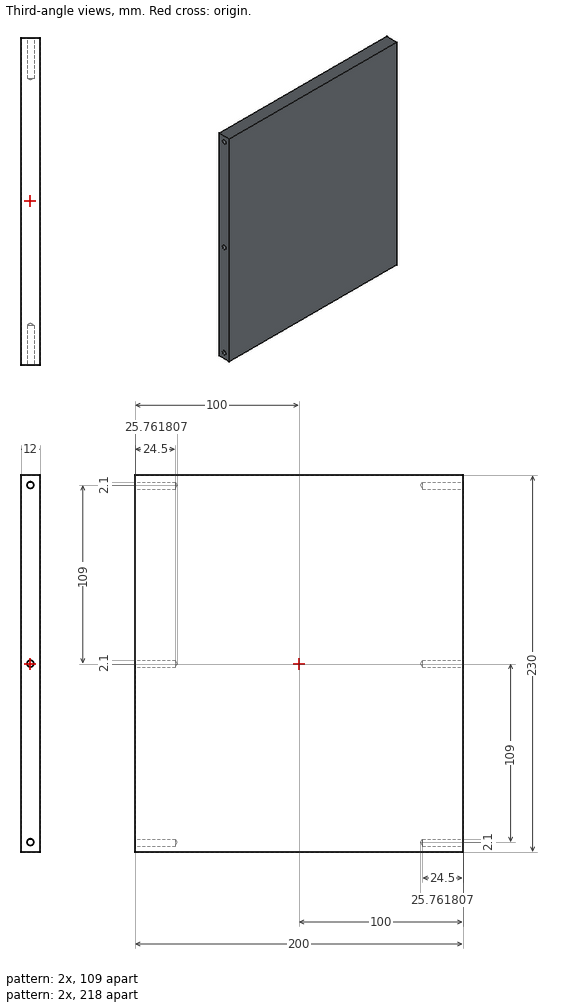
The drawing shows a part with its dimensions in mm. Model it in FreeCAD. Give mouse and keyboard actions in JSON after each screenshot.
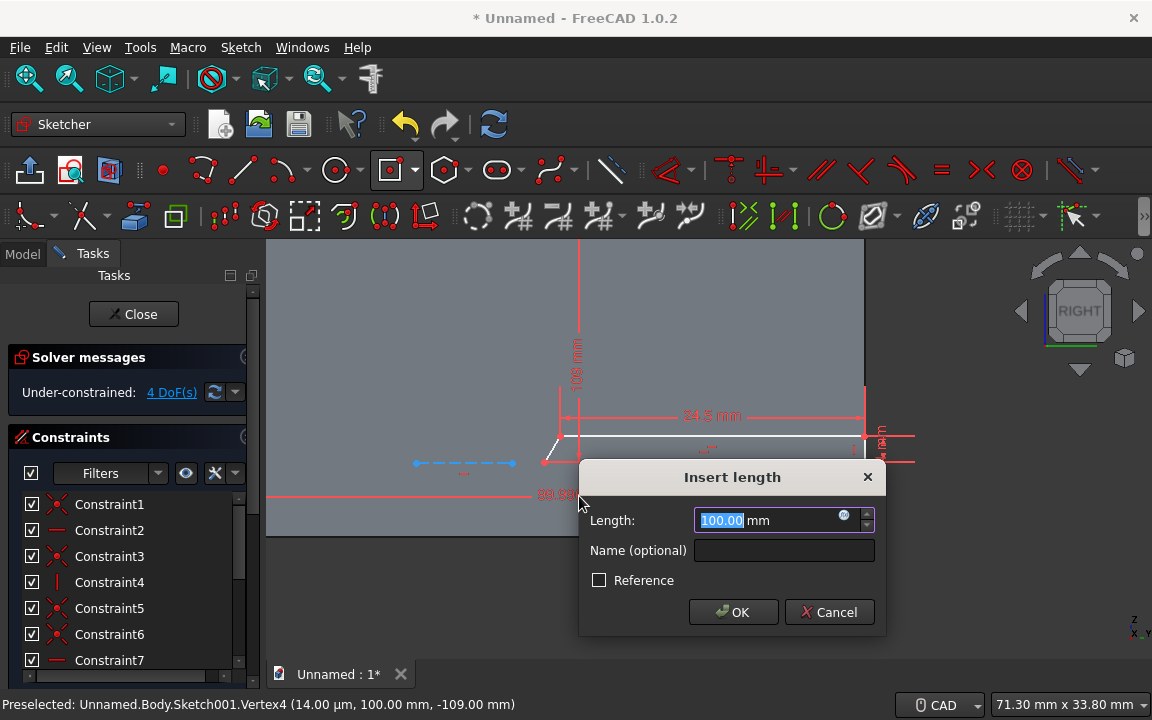
{"action": "type", "text": "100"}
{"action": "key", "text": "Return"}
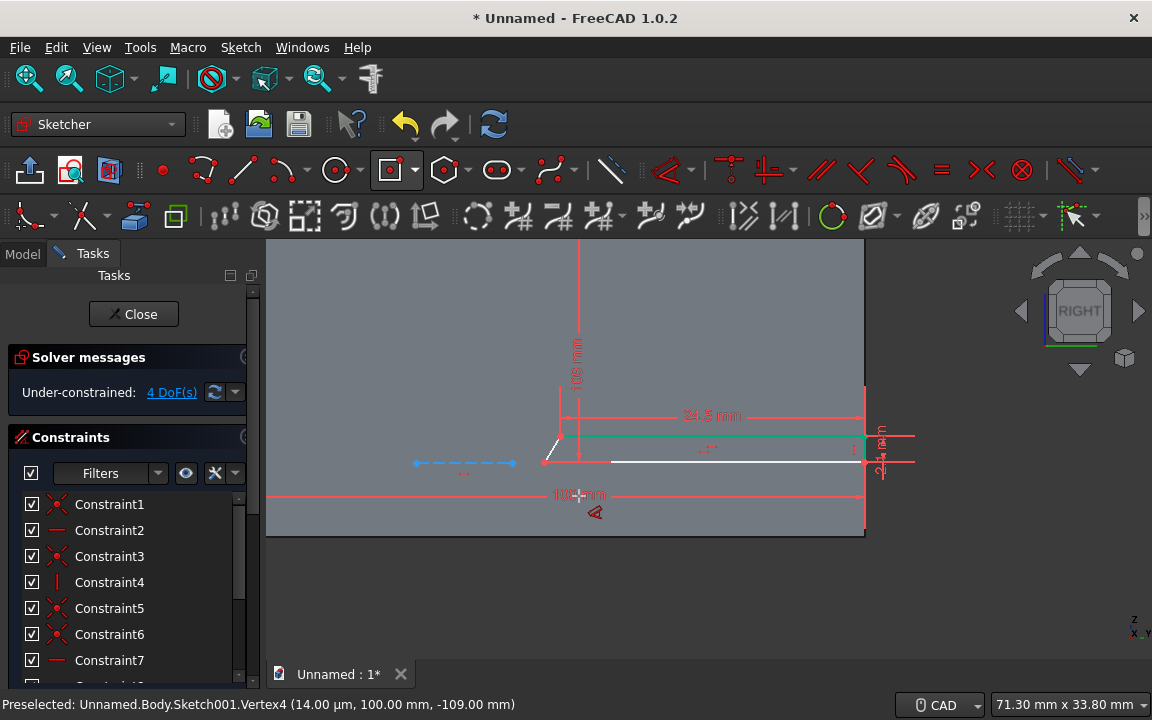
{"action": "left_click", "coordinate": [513, 463]}
{"action": "left_click", "coordinate": [547, 320]}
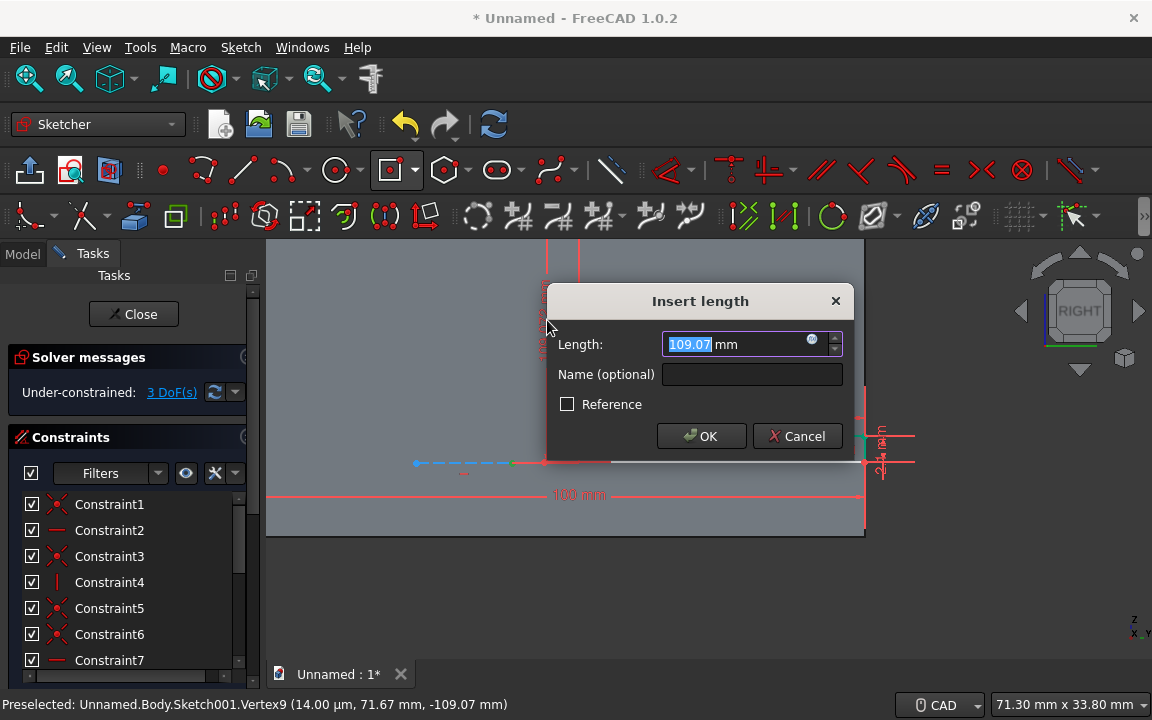
{"action": "type", "text": "109"}
{"action": "key", "text": "Return"}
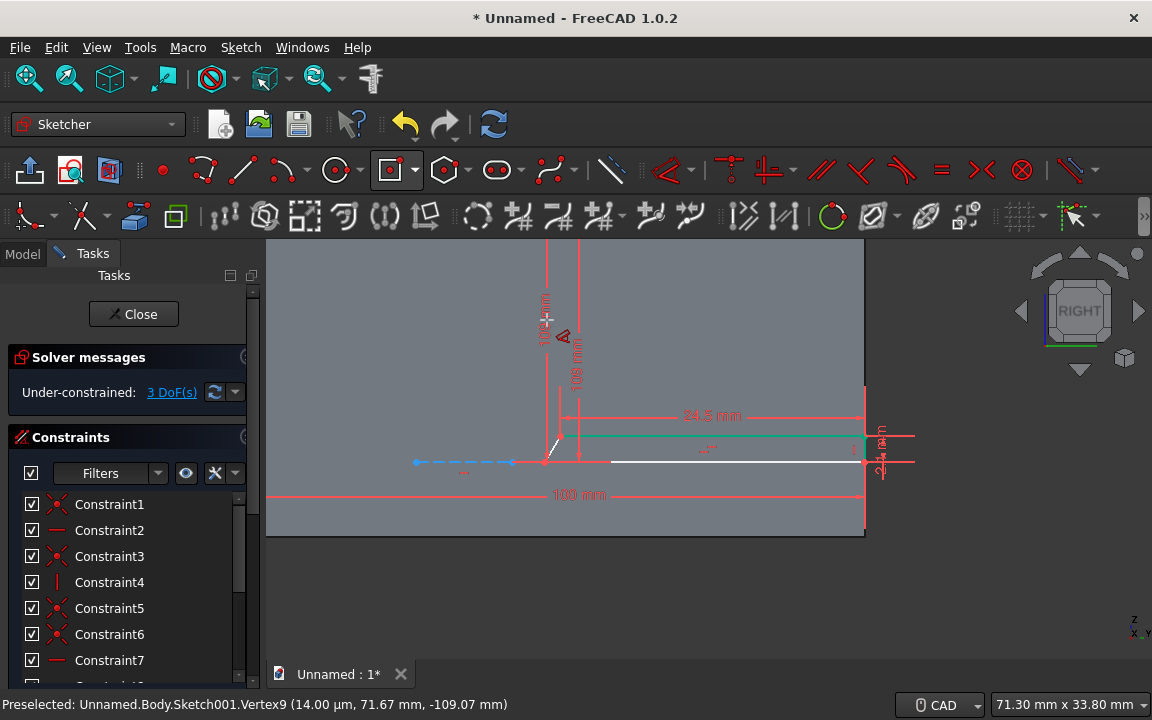
{"action": "left_click", "coordinate": [641, 462]}
{"action": "left_click", "coordinate": [705, 496]}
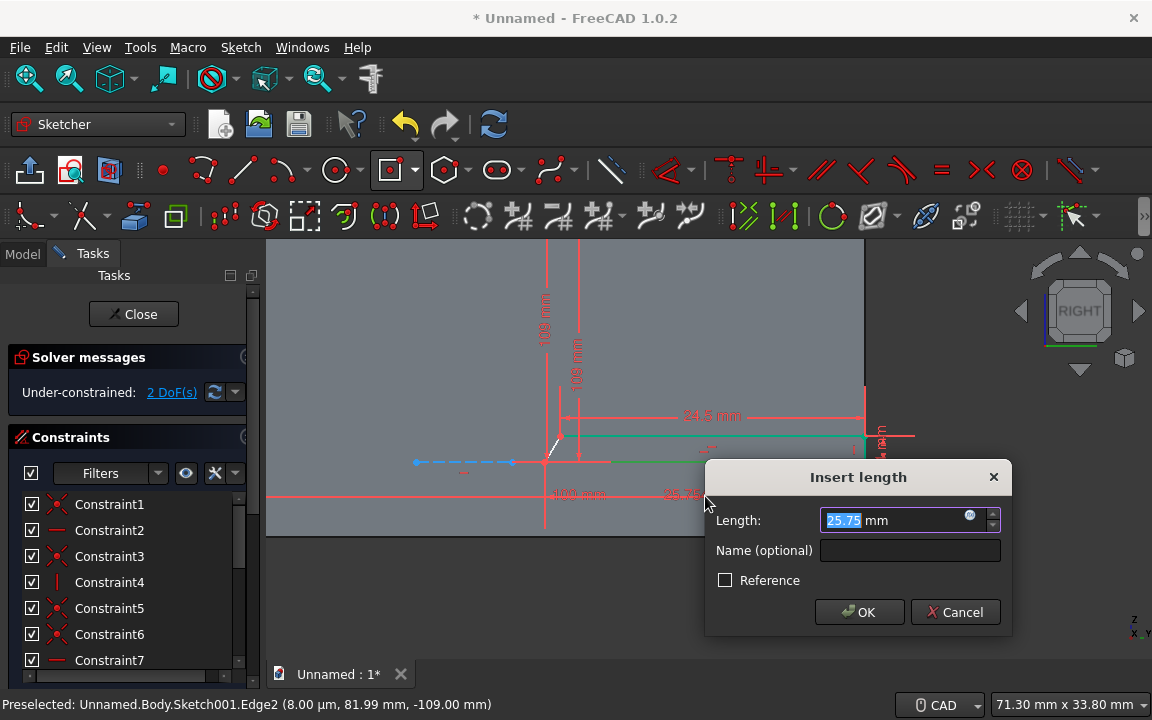
{"action": "type", "text": "25.761807"}
{"action": "key", "text": "Return"}
{"action": "key", "text": "Escape"}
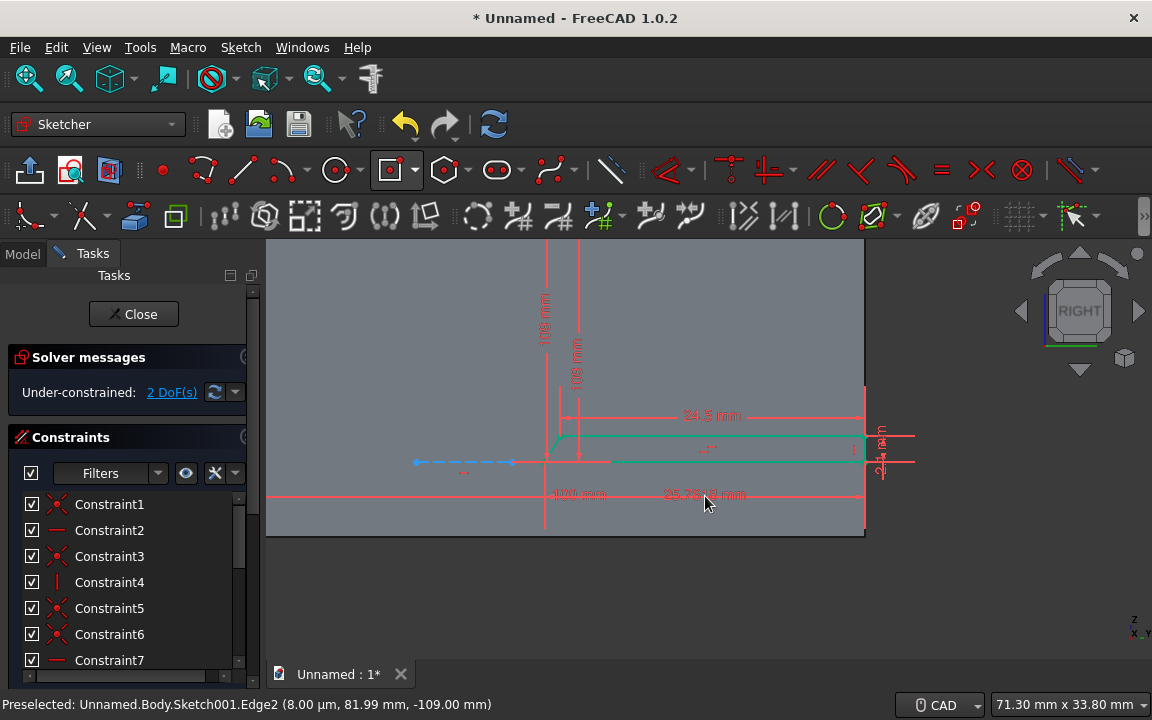
{"action": "left_click", "coordinate": [134, 314]}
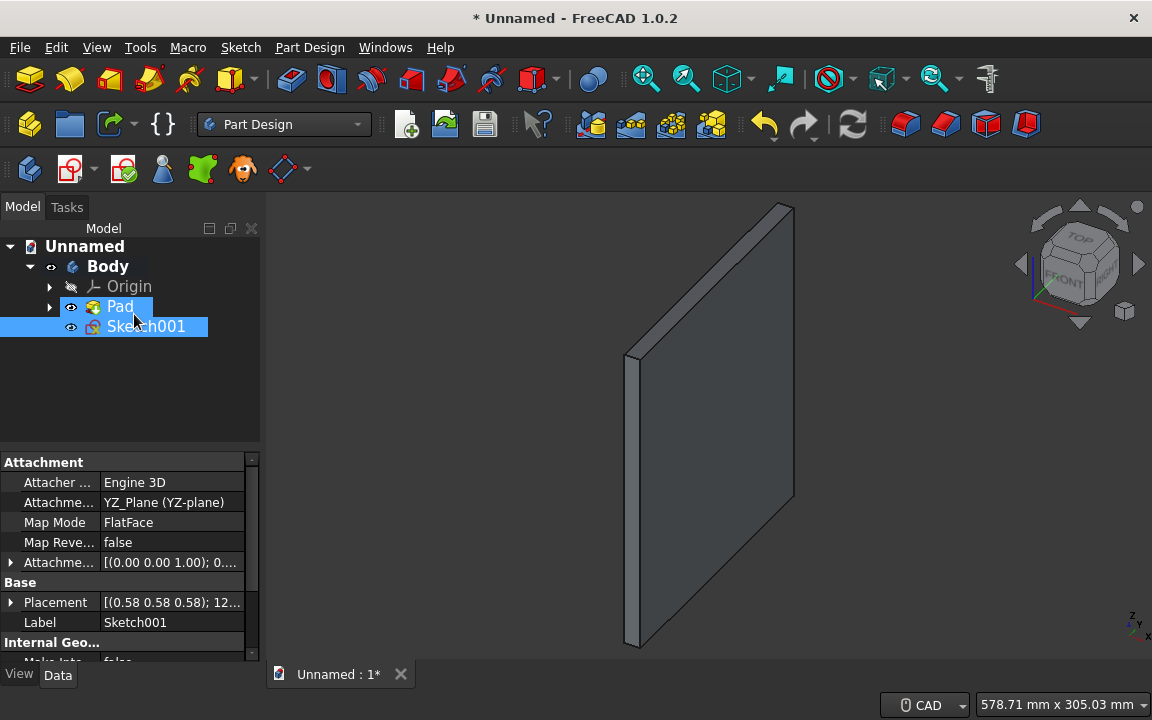
{"action": "left_click", "coordinate": [372, 80]}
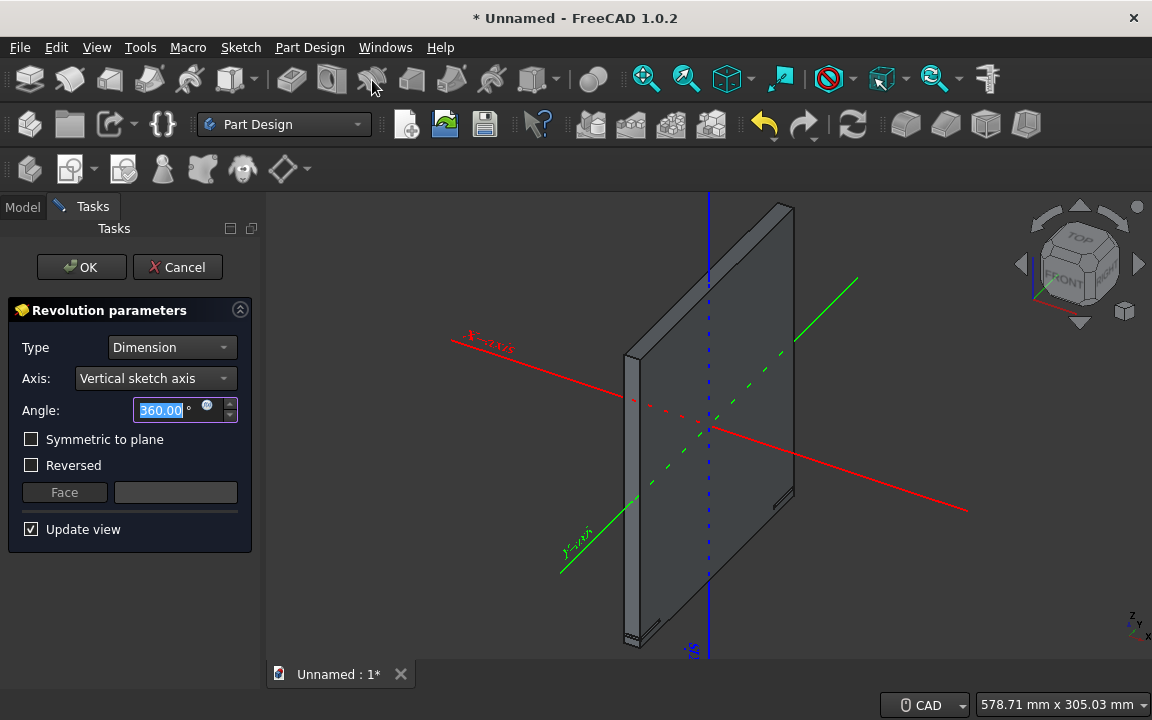
{"action": "left_click", "coordinate": [156, 378]}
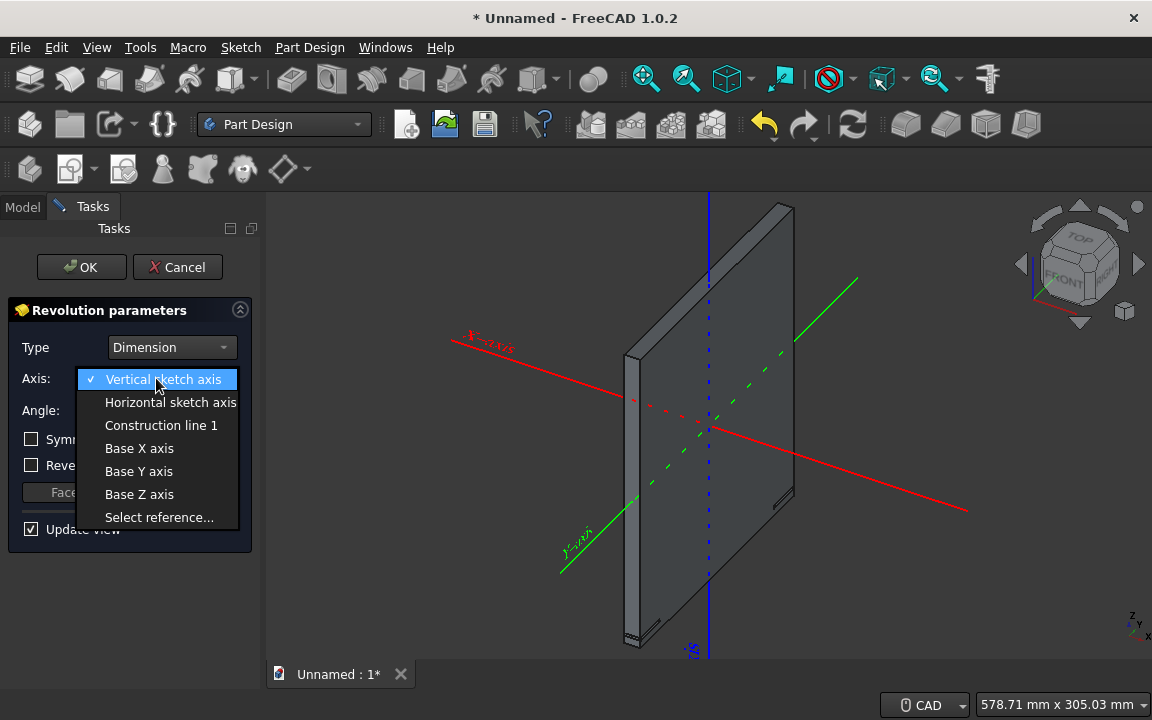
{"action": "left_click", "coordinate": [156, 426]}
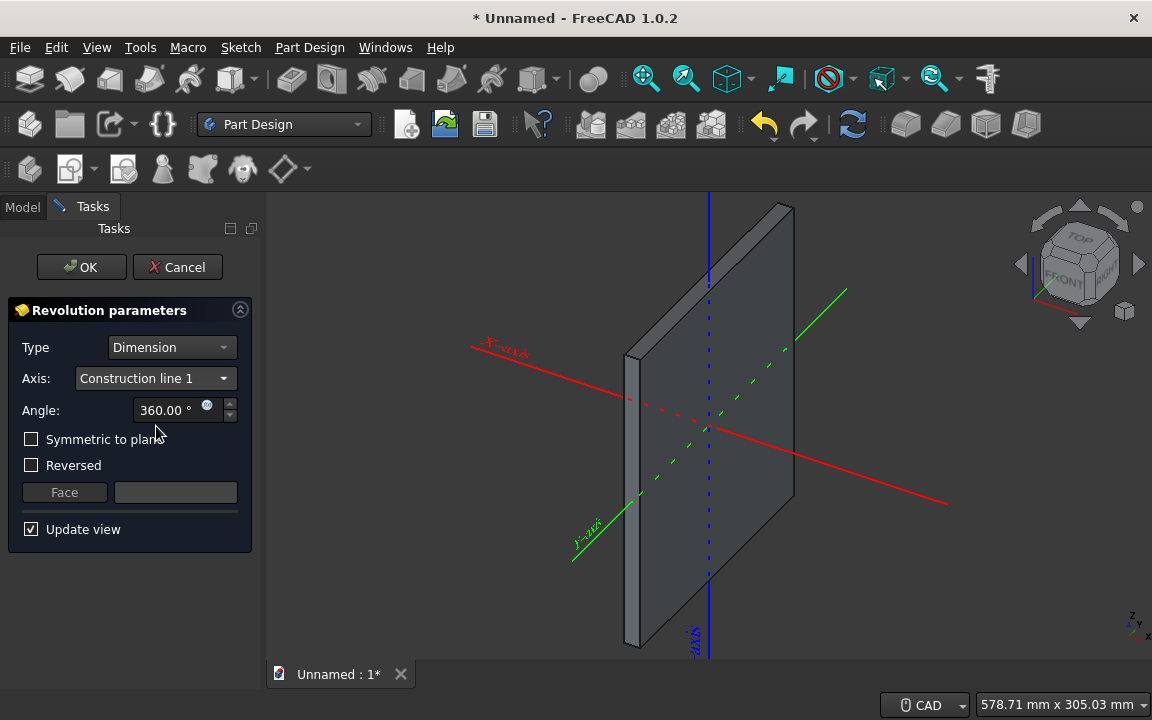
{"action": "left_click", "coordinate": [82, 267]}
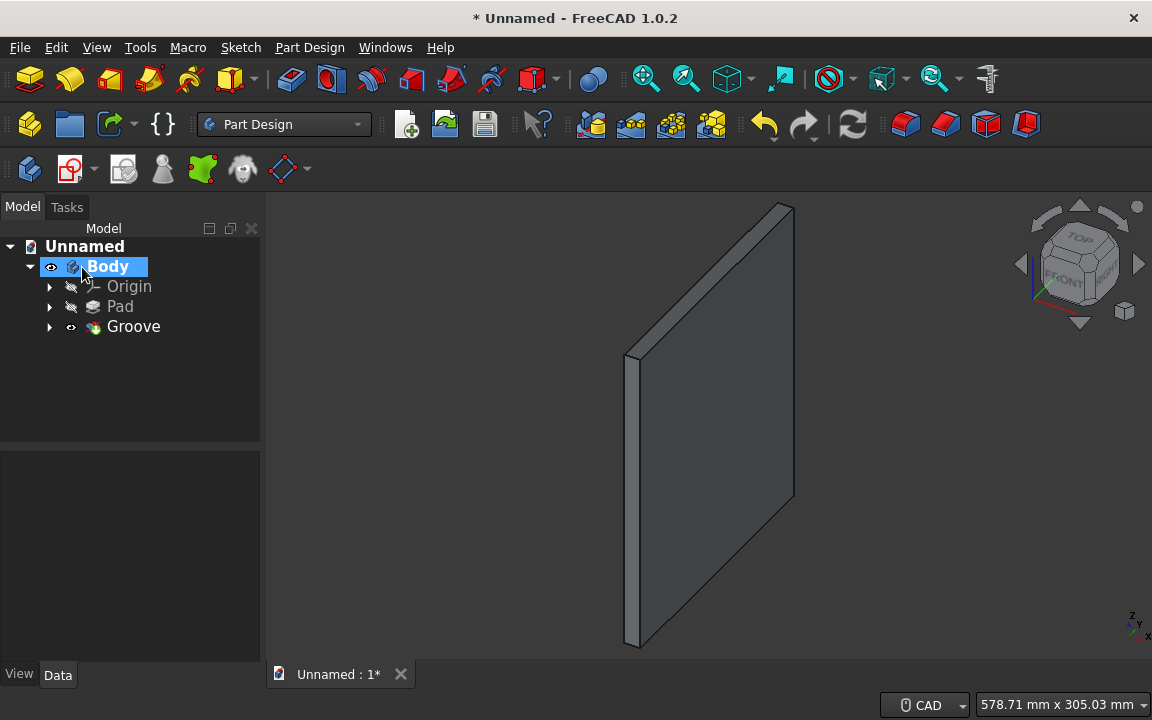
{"action": "left_click", "coordinate": [116, 327]}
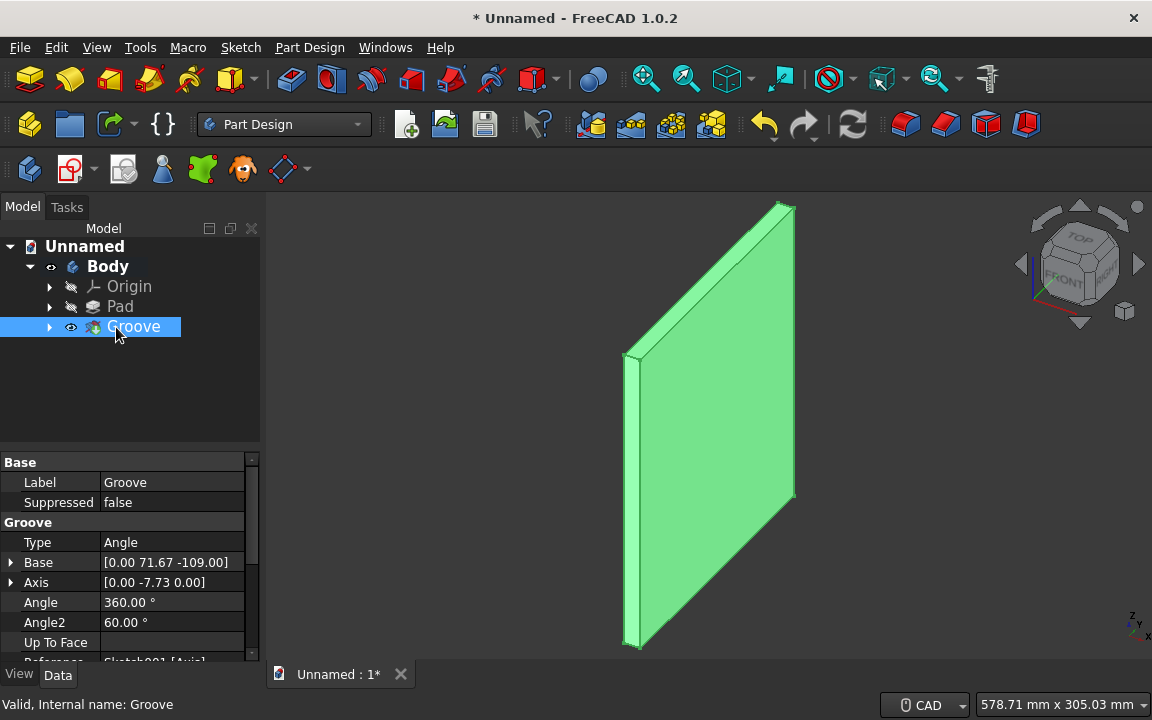
{"action": "left_click", "coordinate": [632, 124]}